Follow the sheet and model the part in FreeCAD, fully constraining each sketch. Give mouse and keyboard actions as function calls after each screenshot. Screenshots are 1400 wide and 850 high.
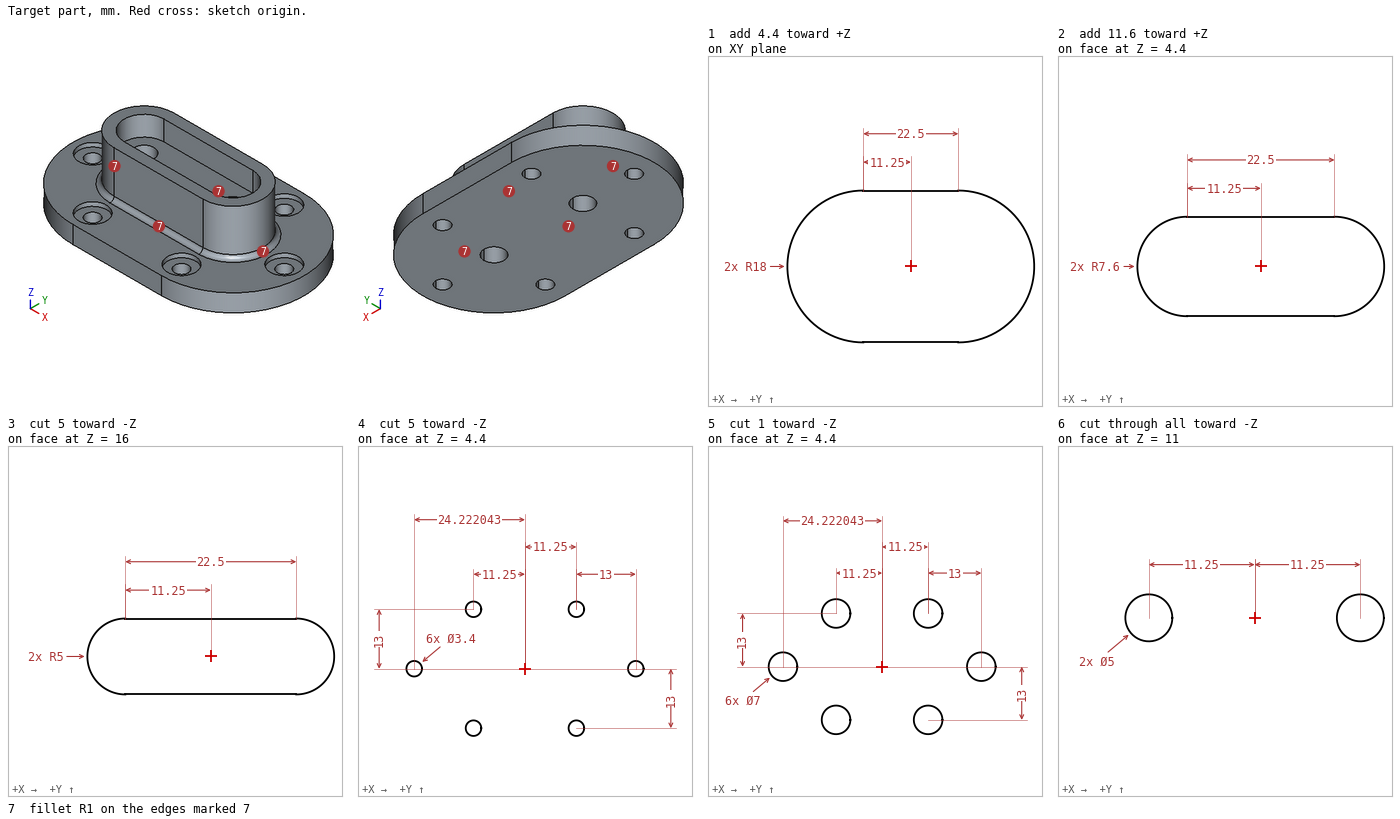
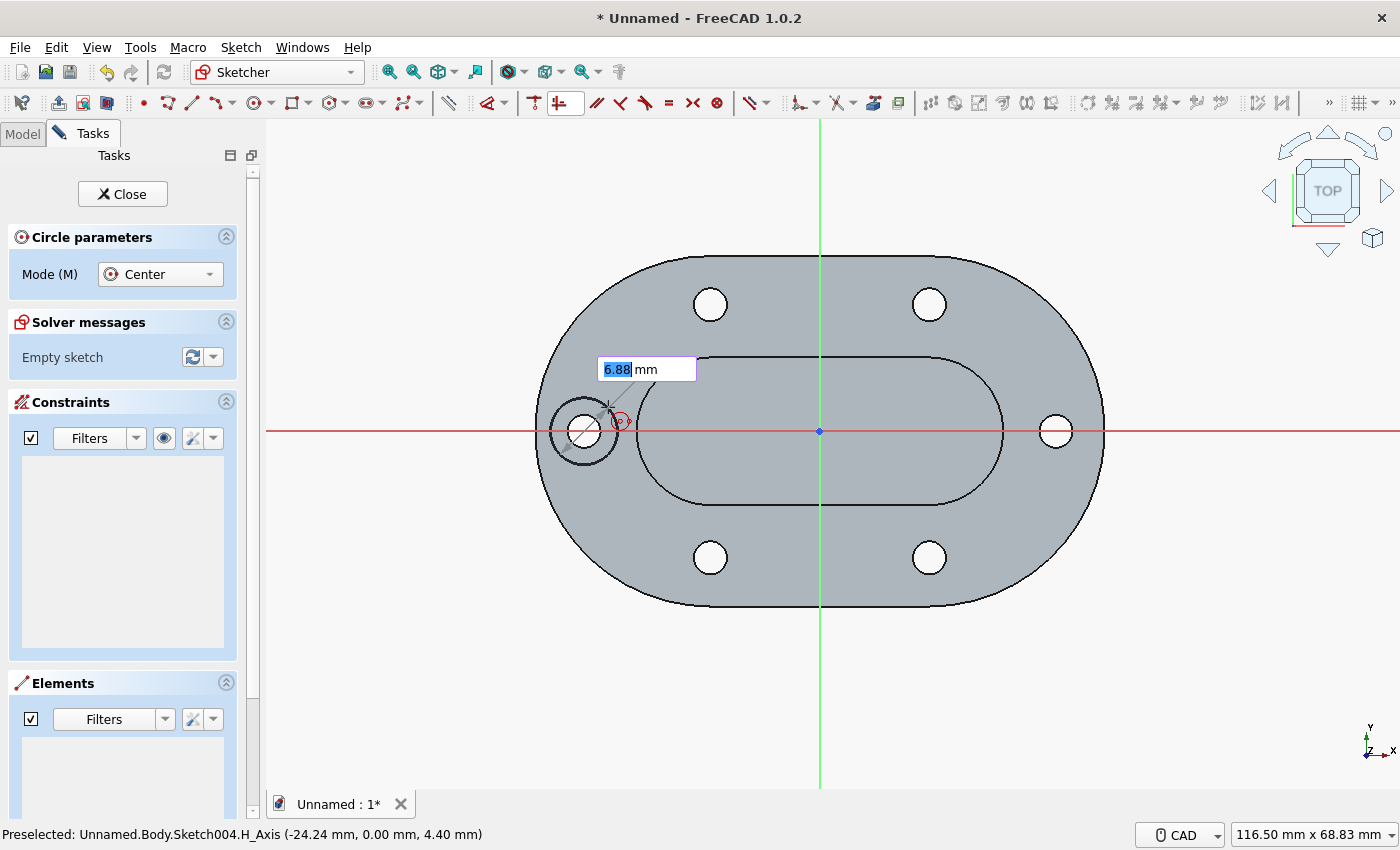
text(7)
key(Return)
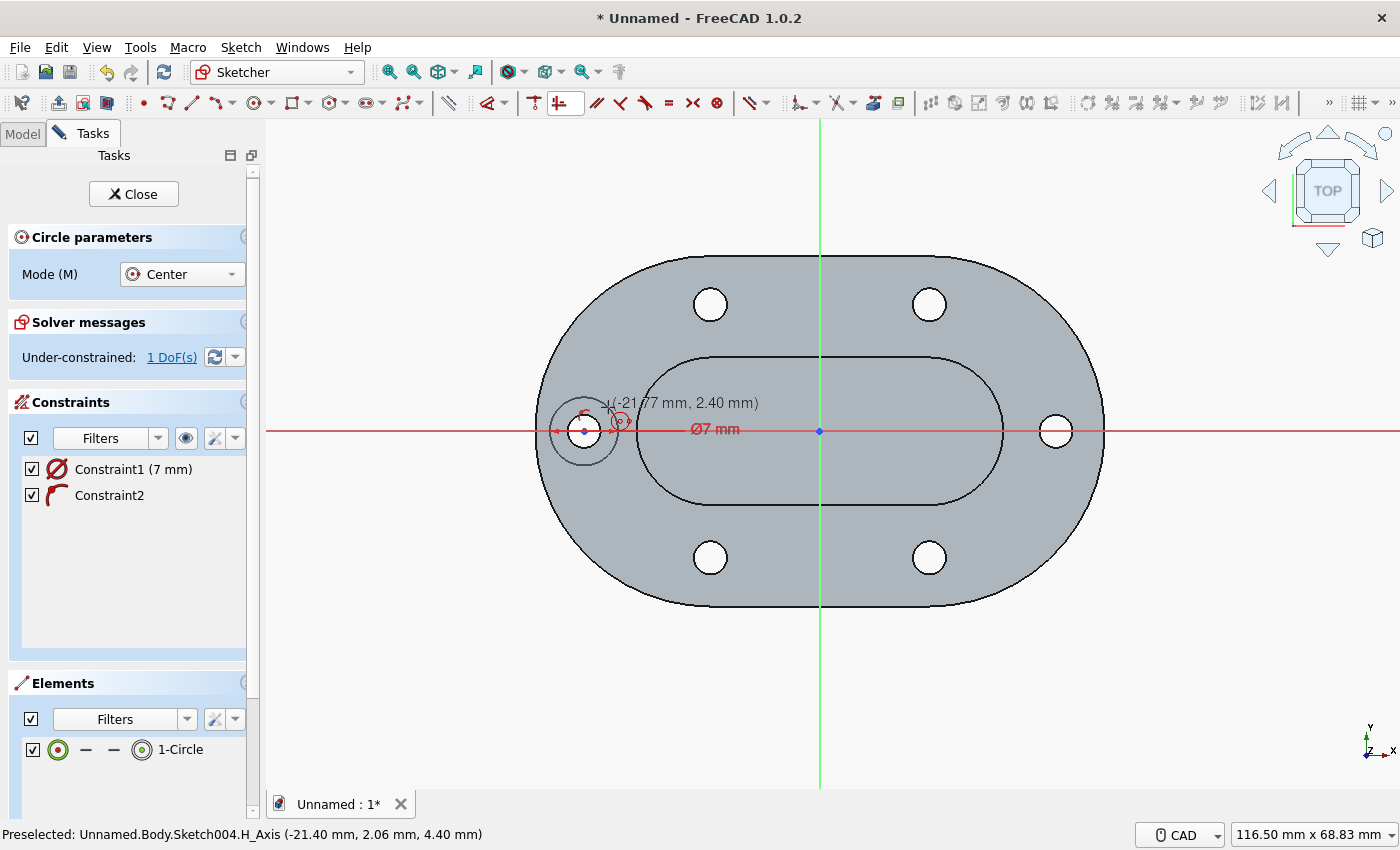
click(710, 305)
move(734, 281)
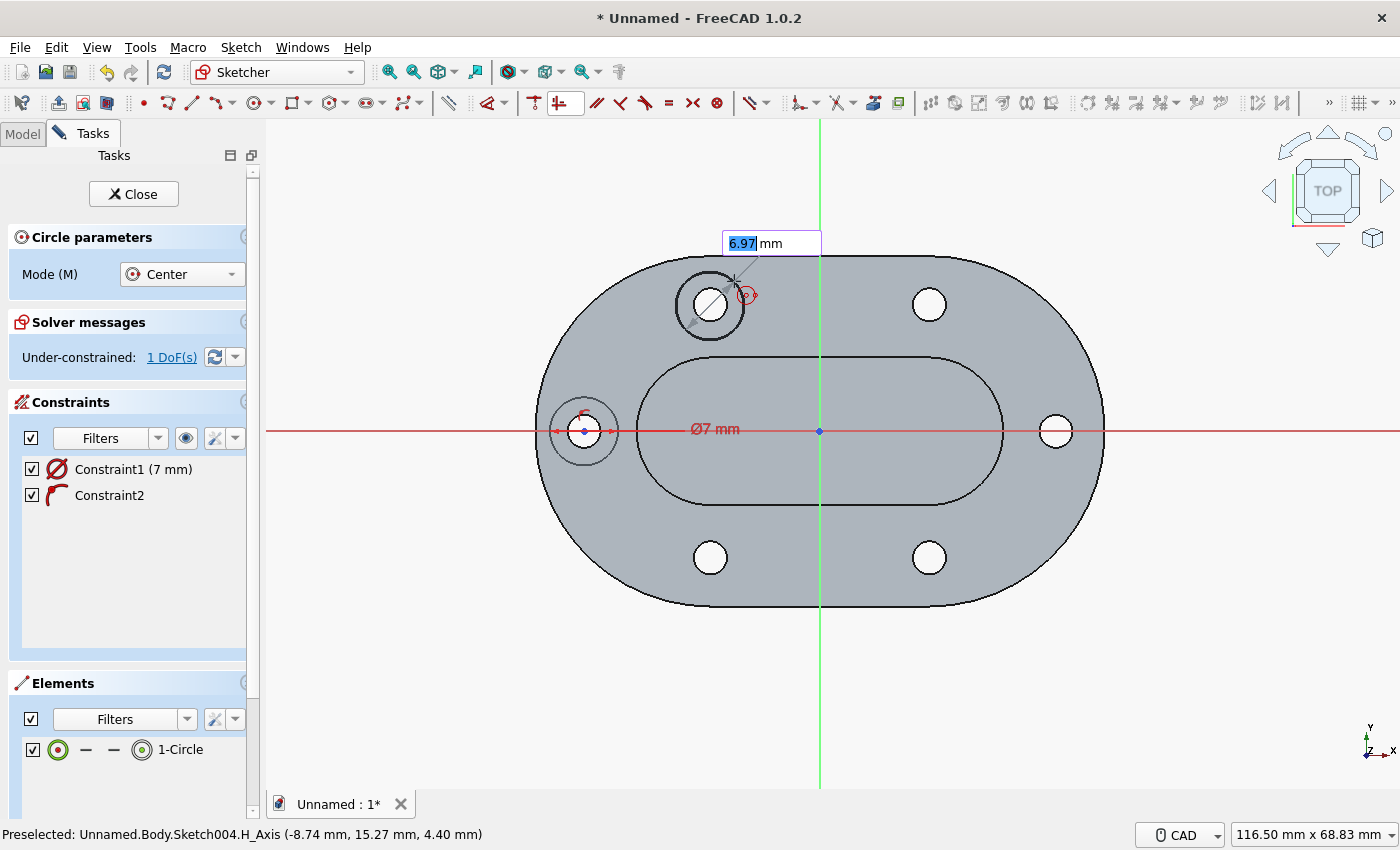
text(7)
key(Return)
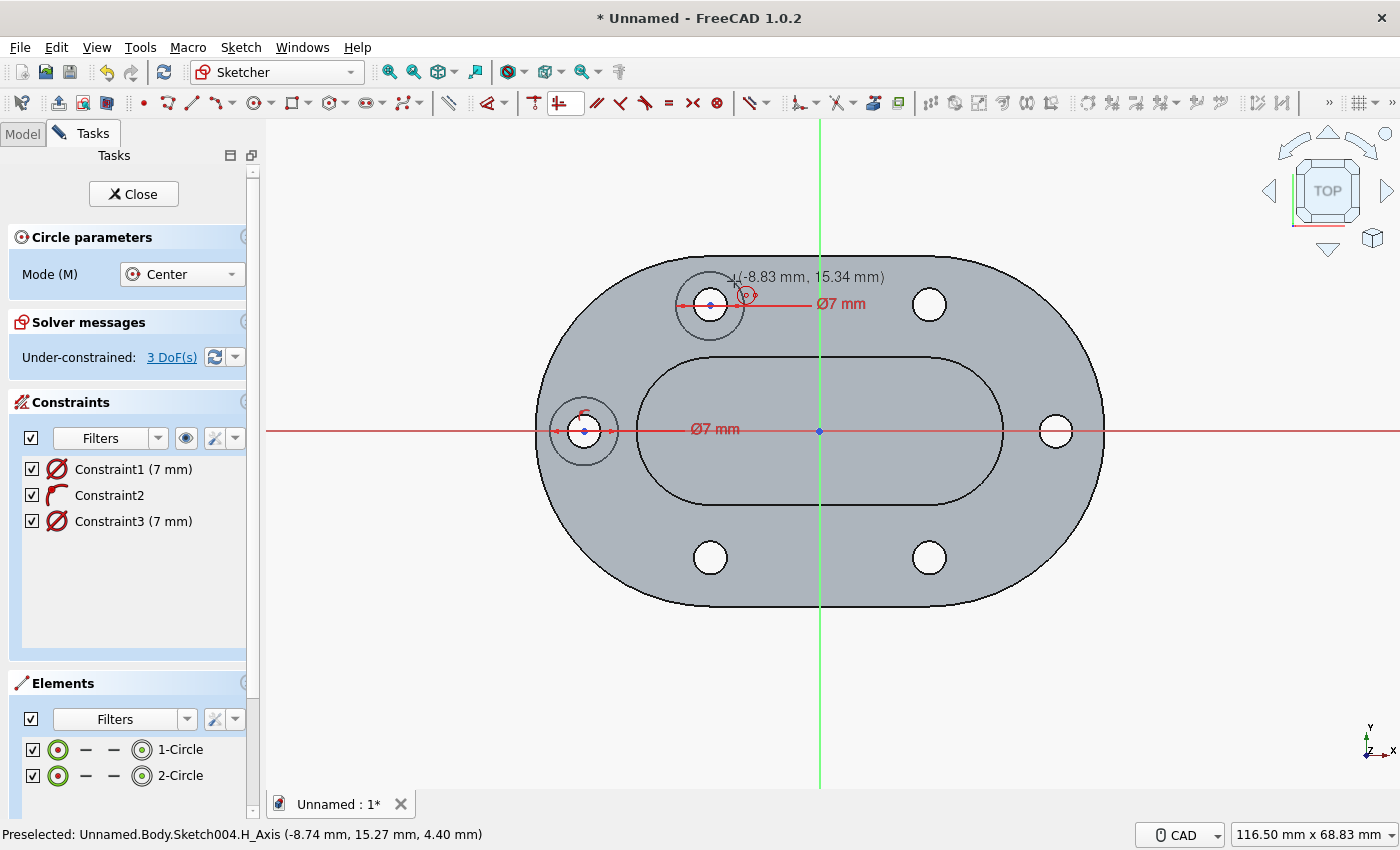
click(929, 305)
move(954, 281)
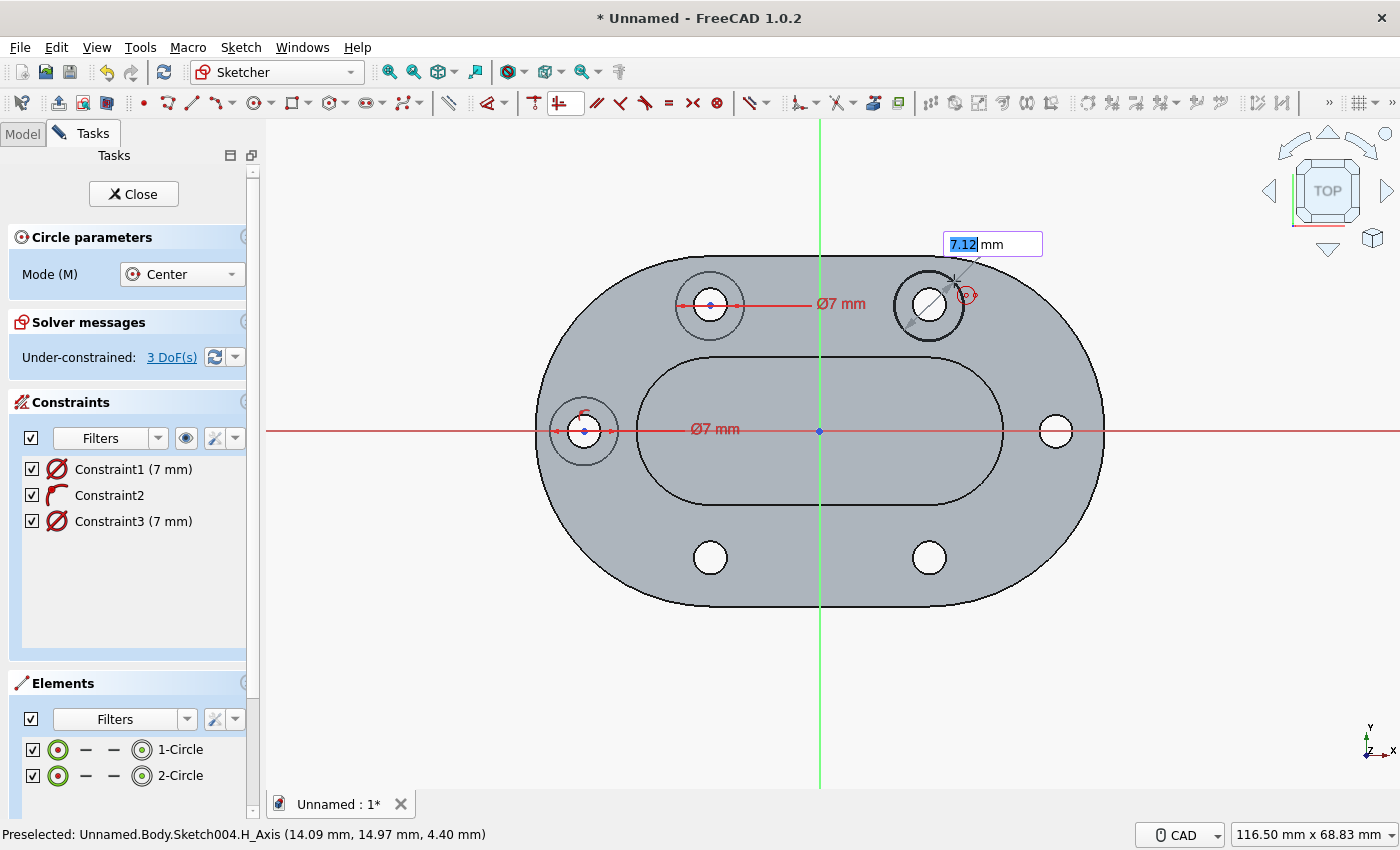
text(7)
key(Return)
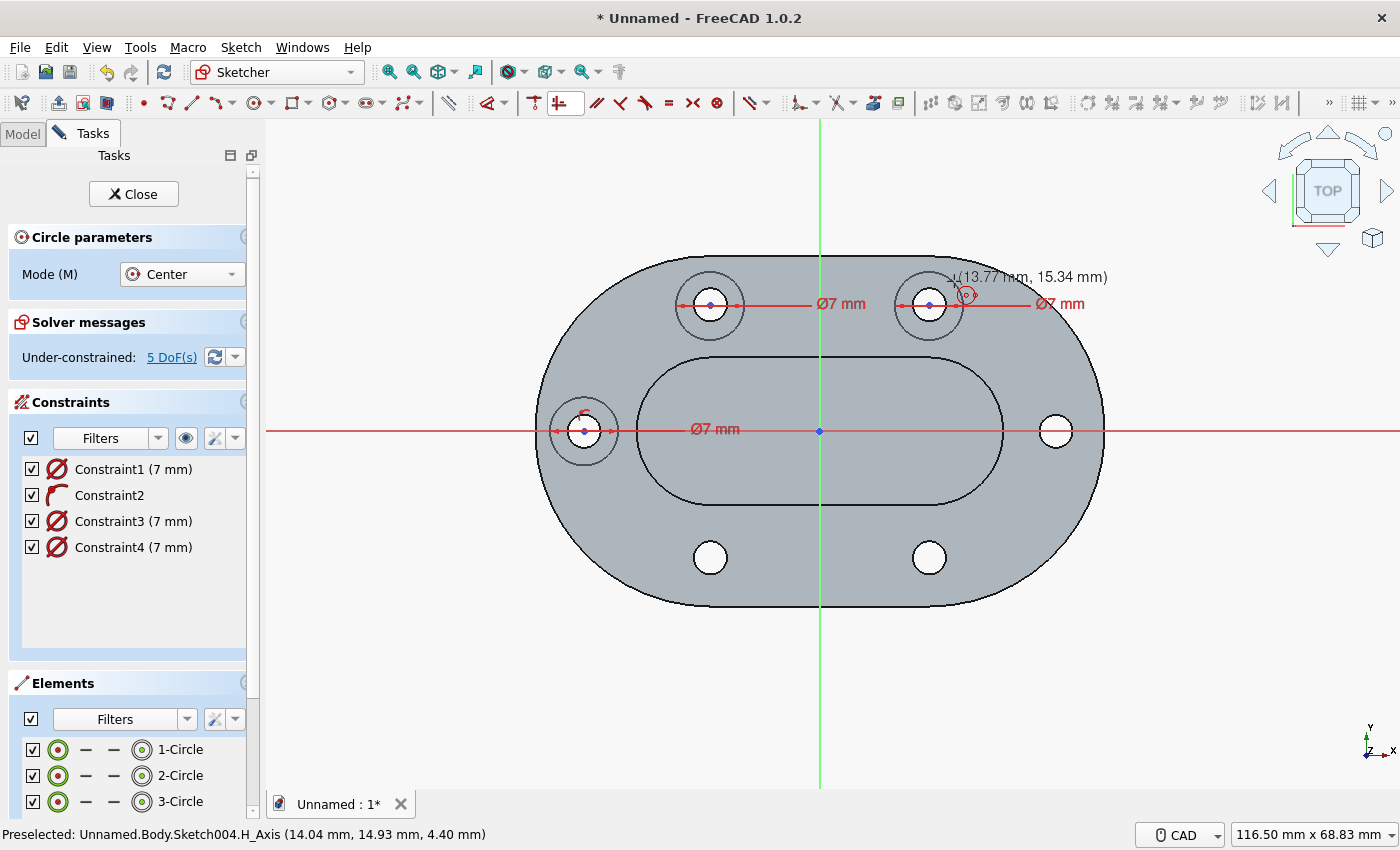
click(1056, 431)
move(1080, 407)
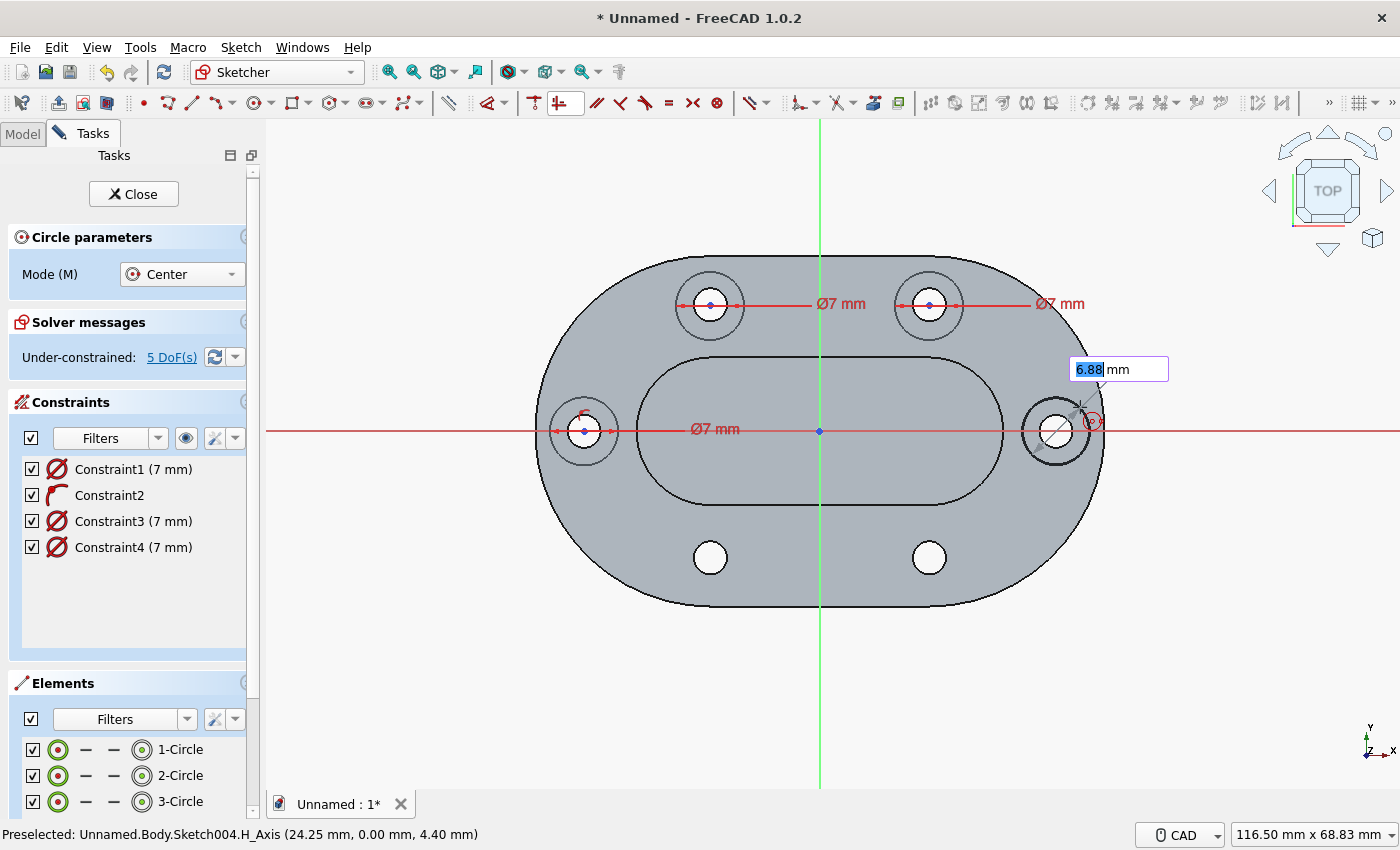
text(7)
key(Return)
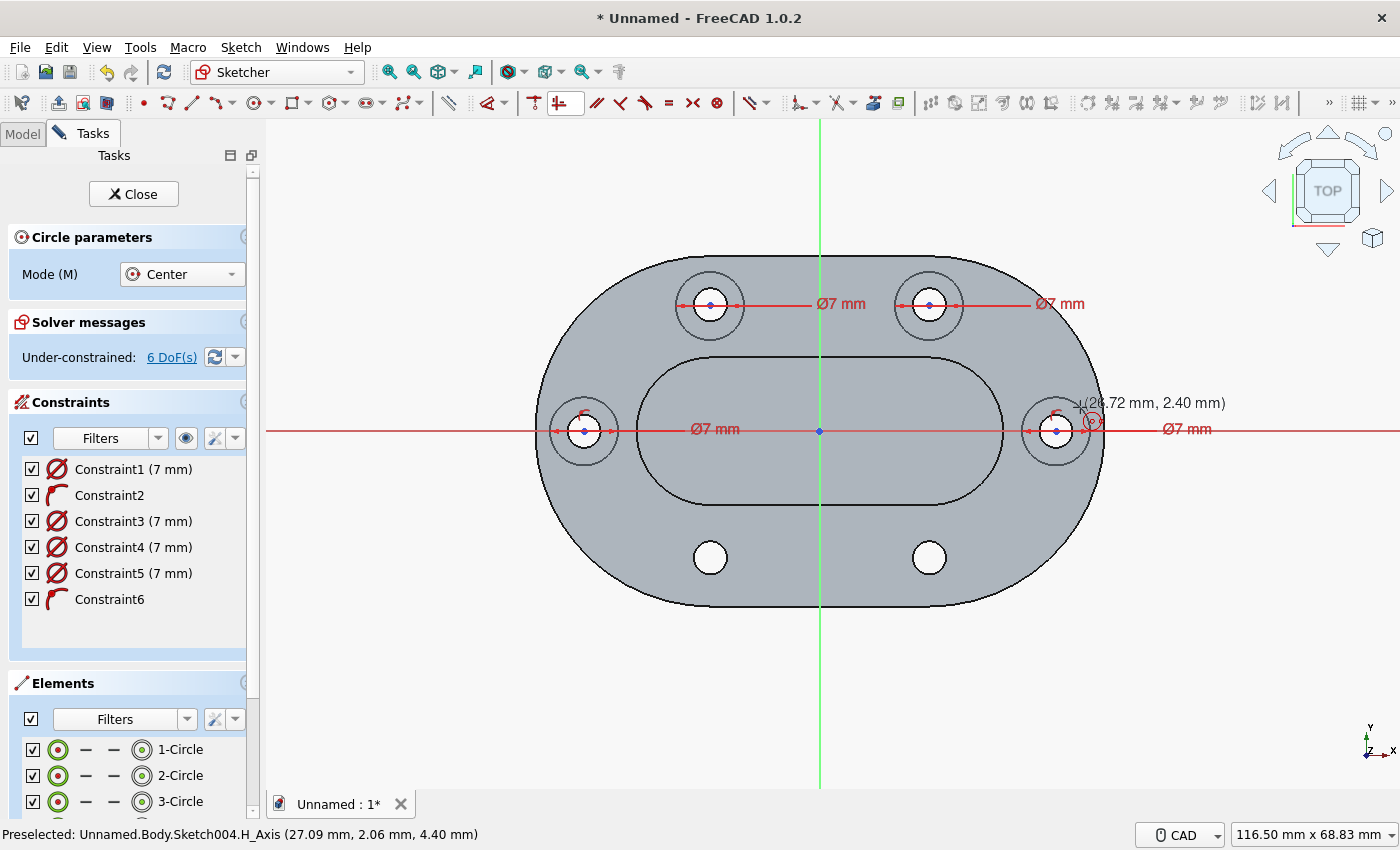
click(929, 558)
move(954, 534)